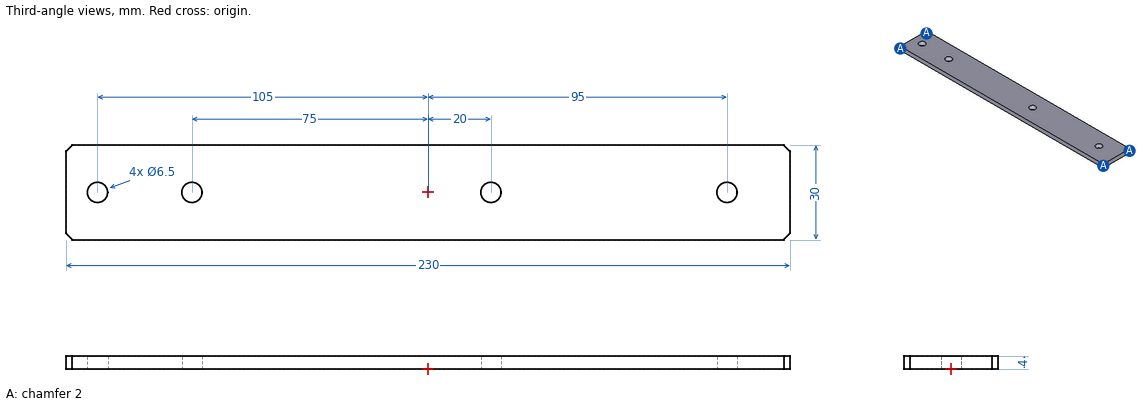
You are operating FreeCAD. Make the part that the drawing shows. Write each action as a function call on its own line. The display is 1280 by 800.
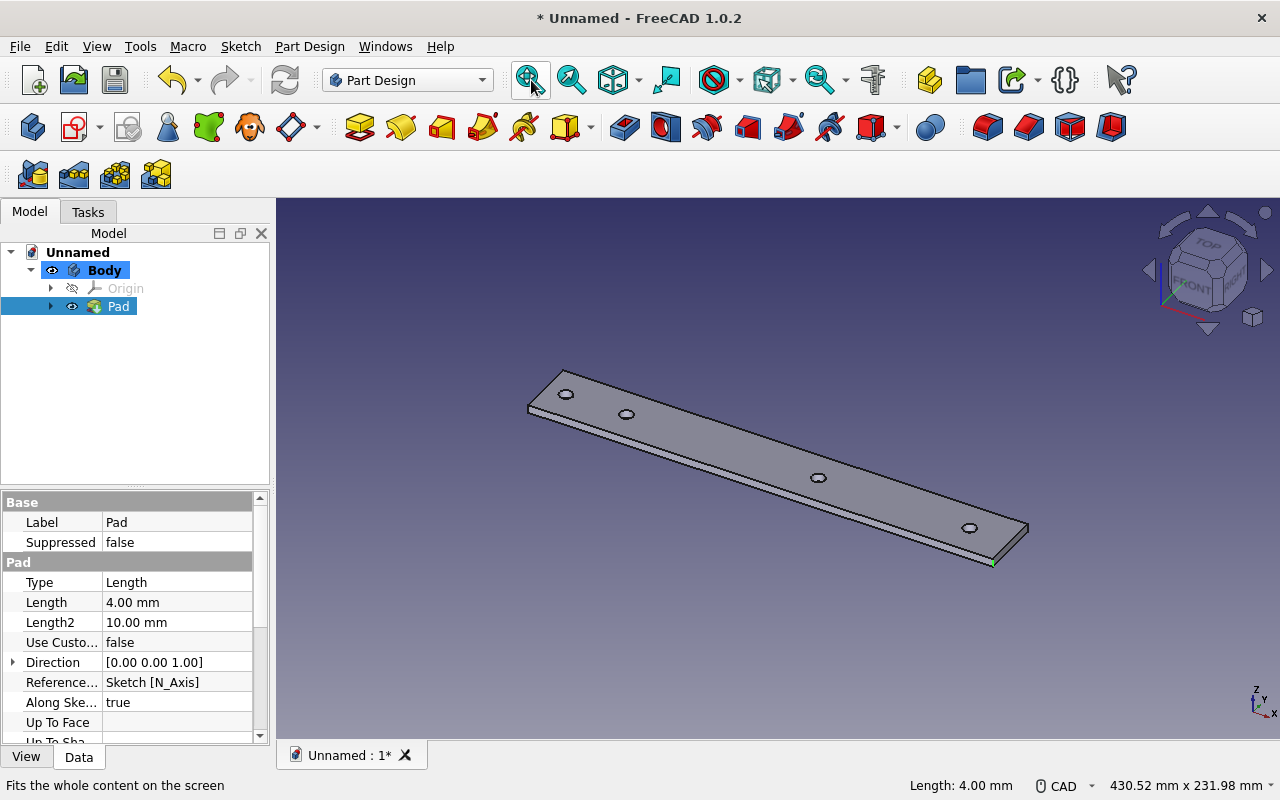
key(0)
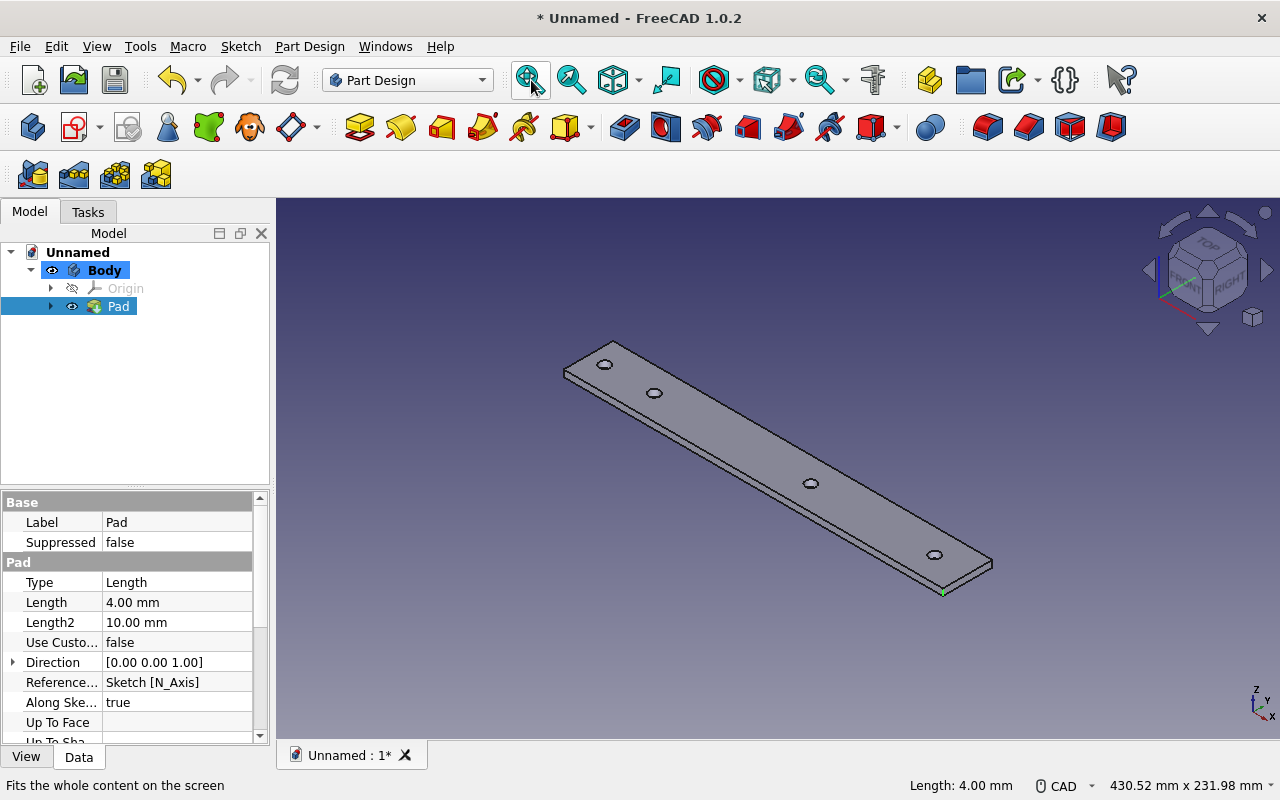
scroll(613, 344, up, 8)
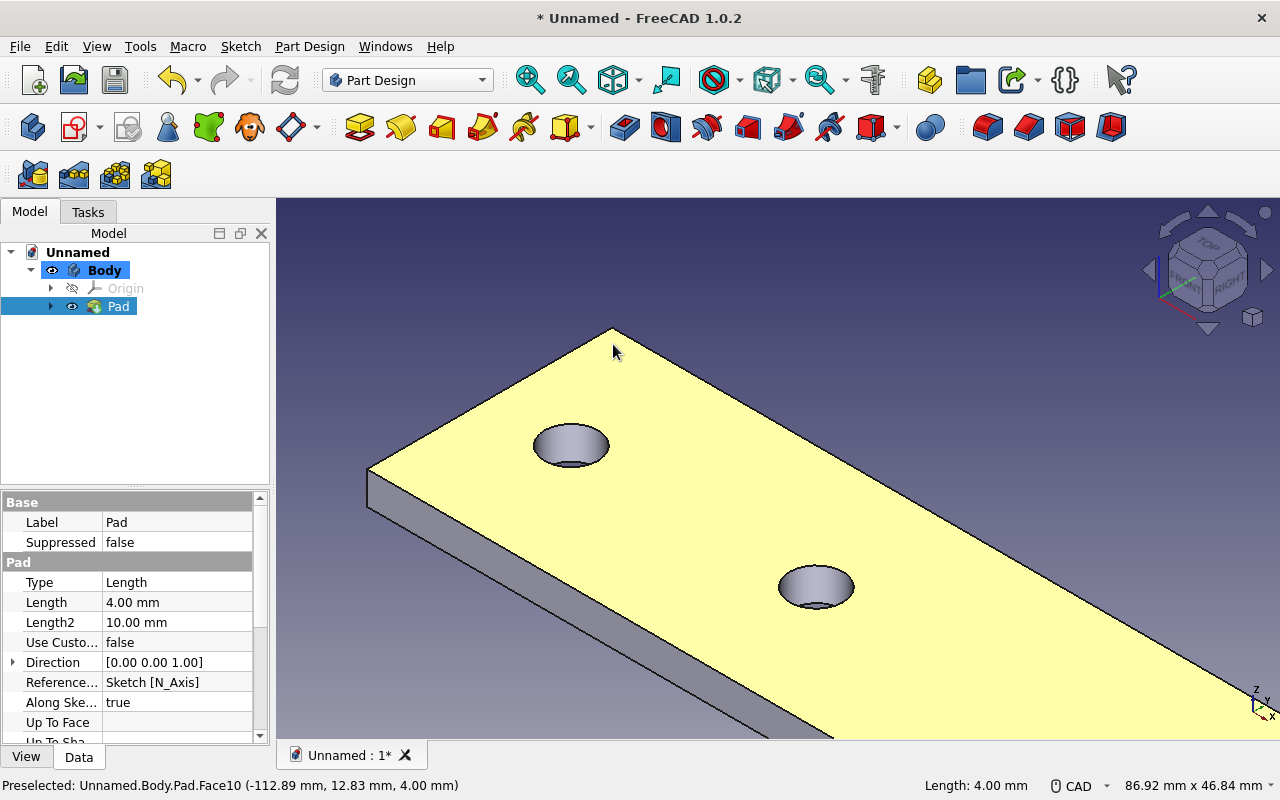
click(531, 80)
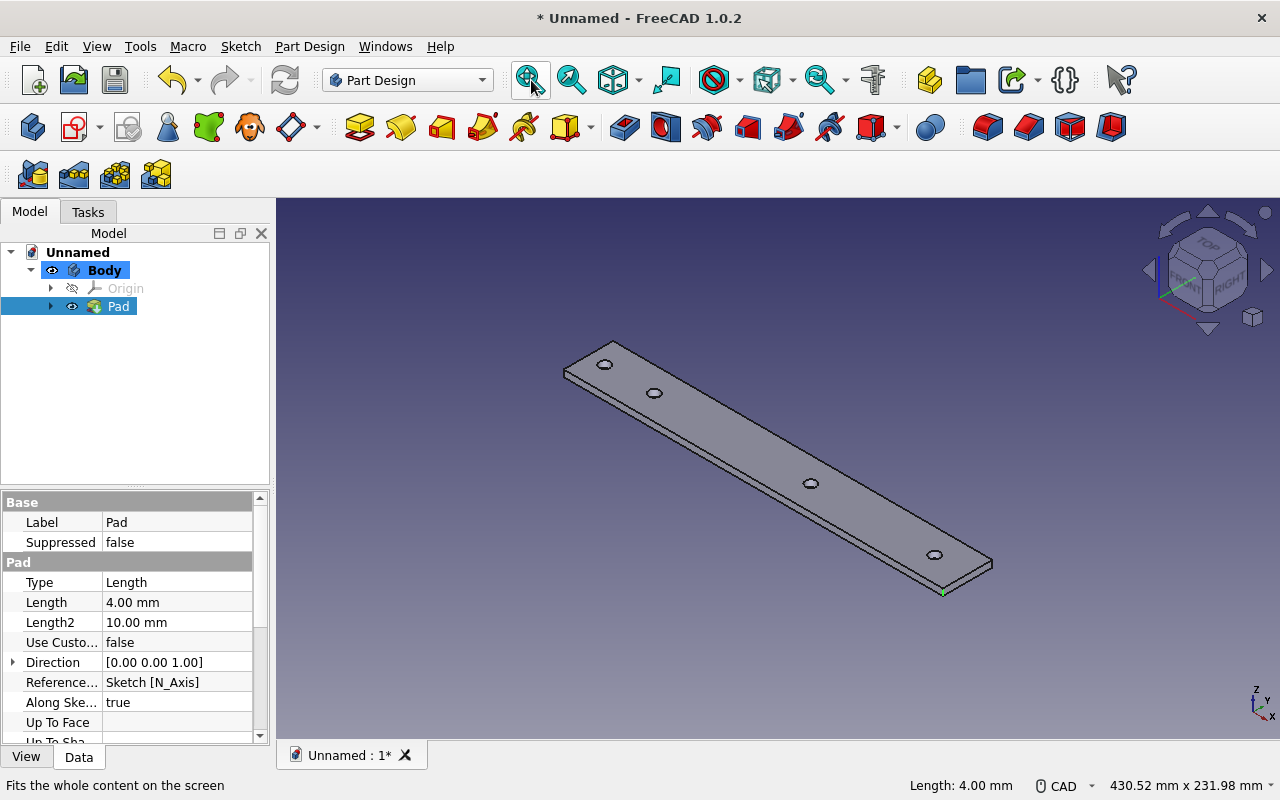
key(2)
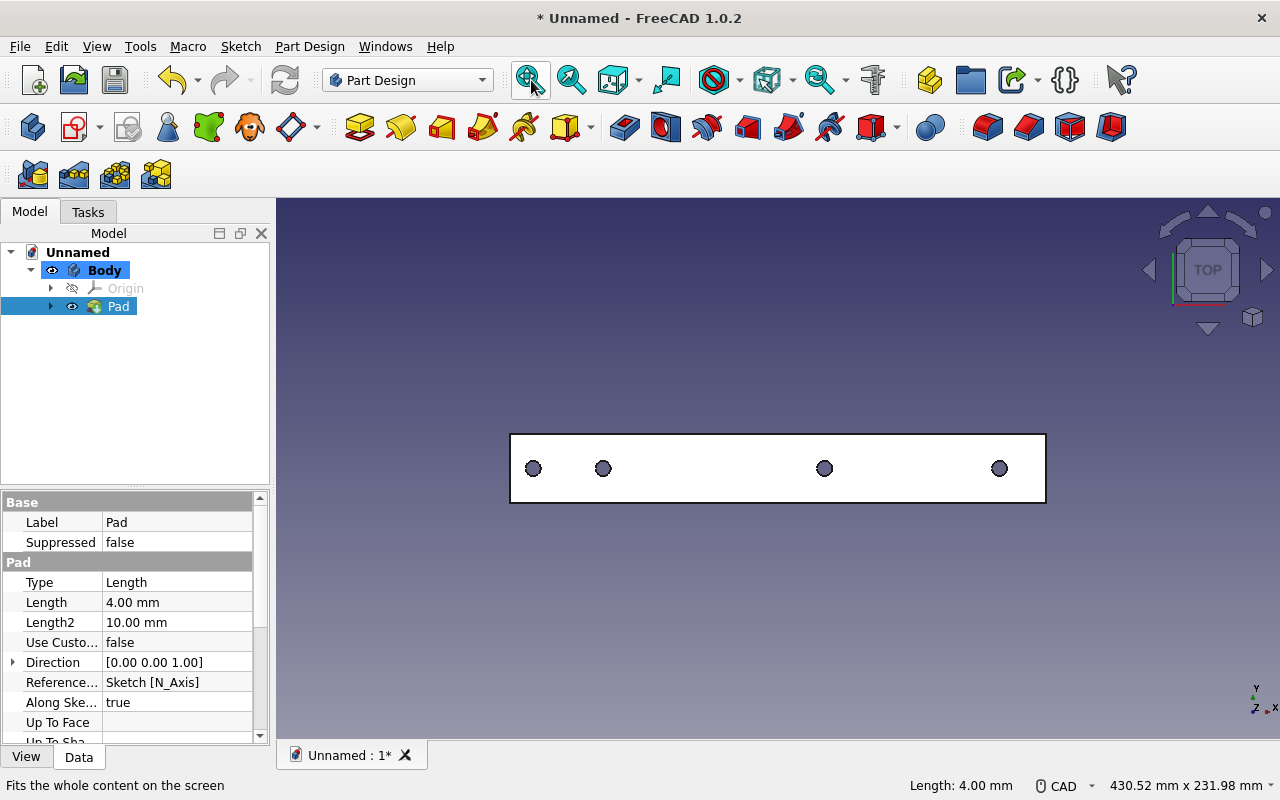
scroll(510, 433, up, 8)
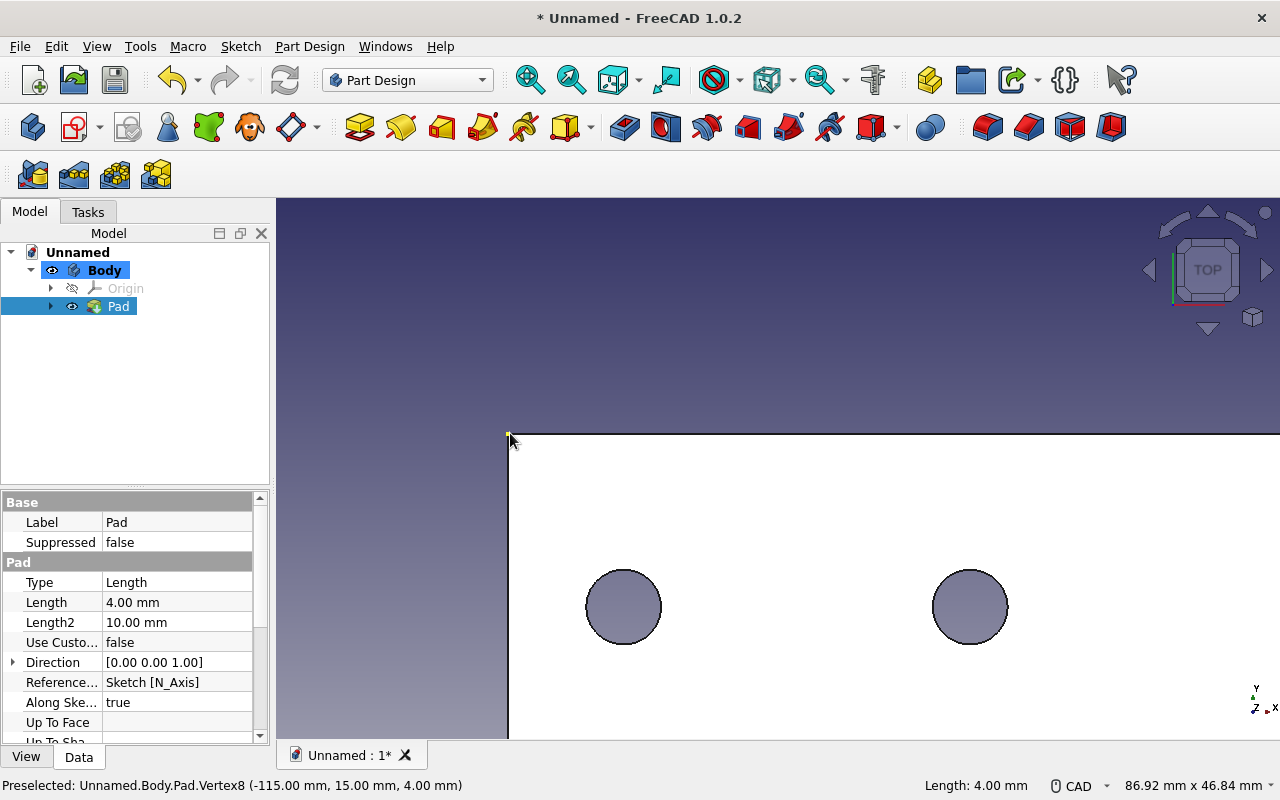
key(v)
key(f)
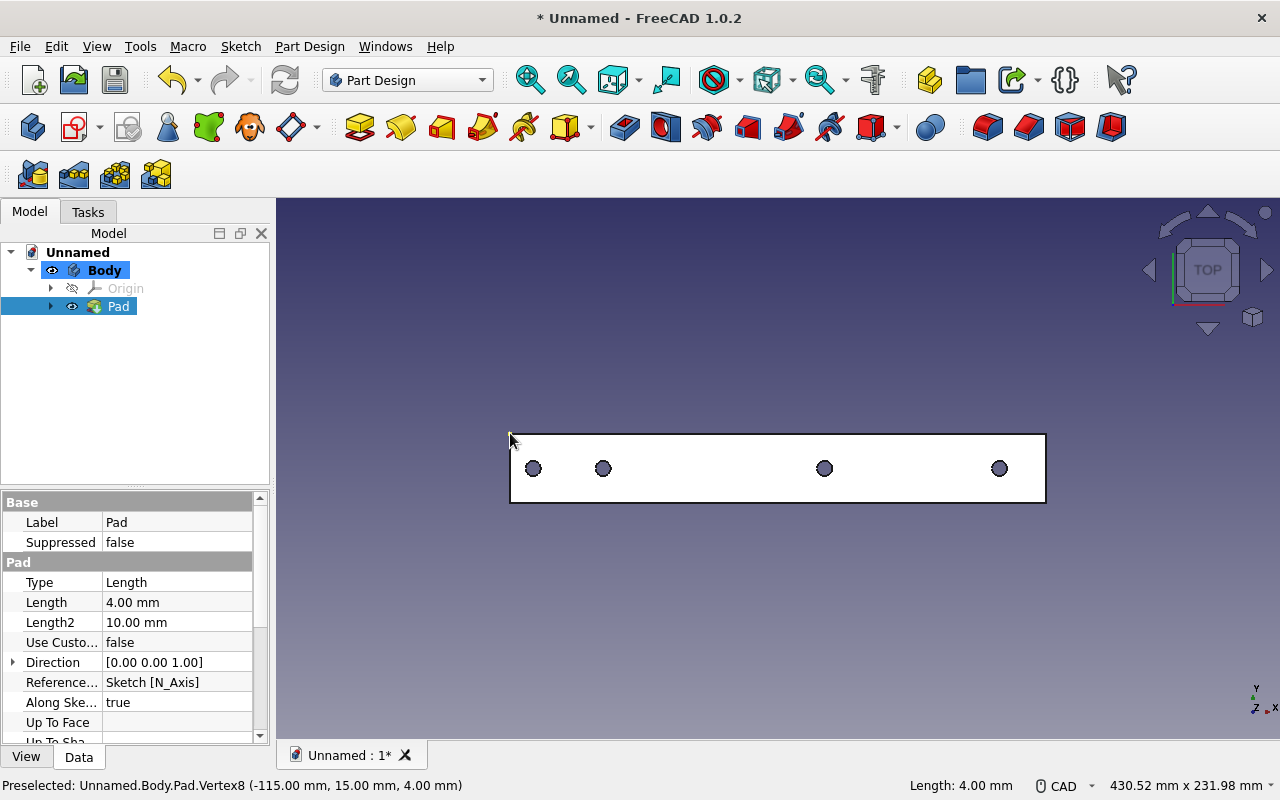
key(1)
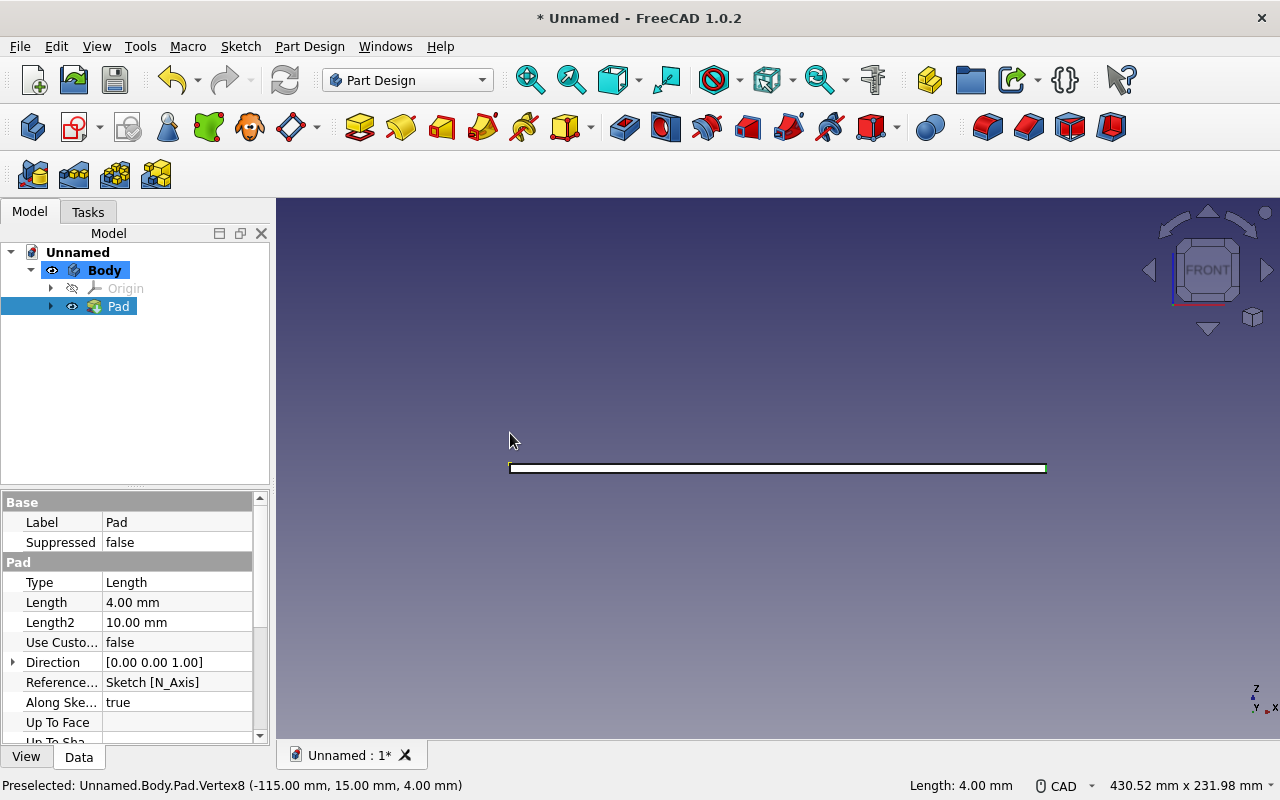
scroll(510, 468, up, 8)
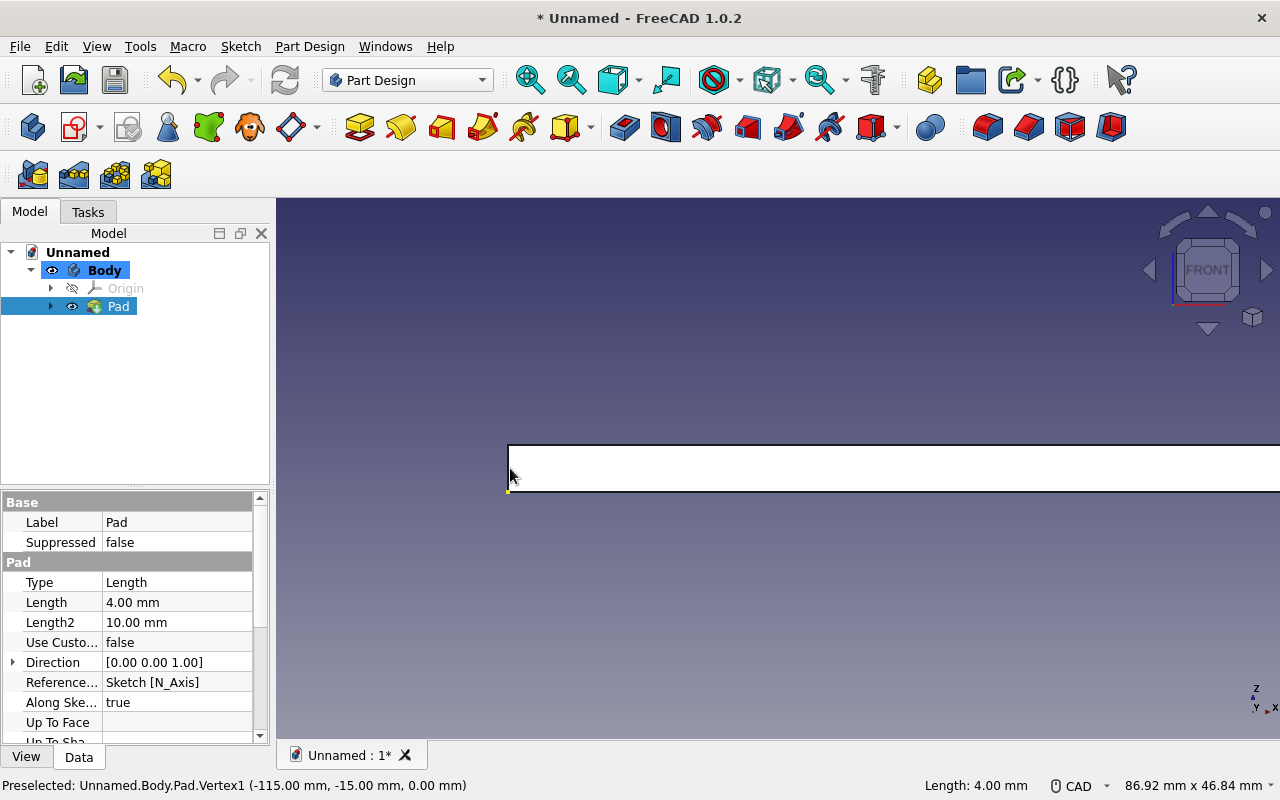
click(508, 468, ctrl)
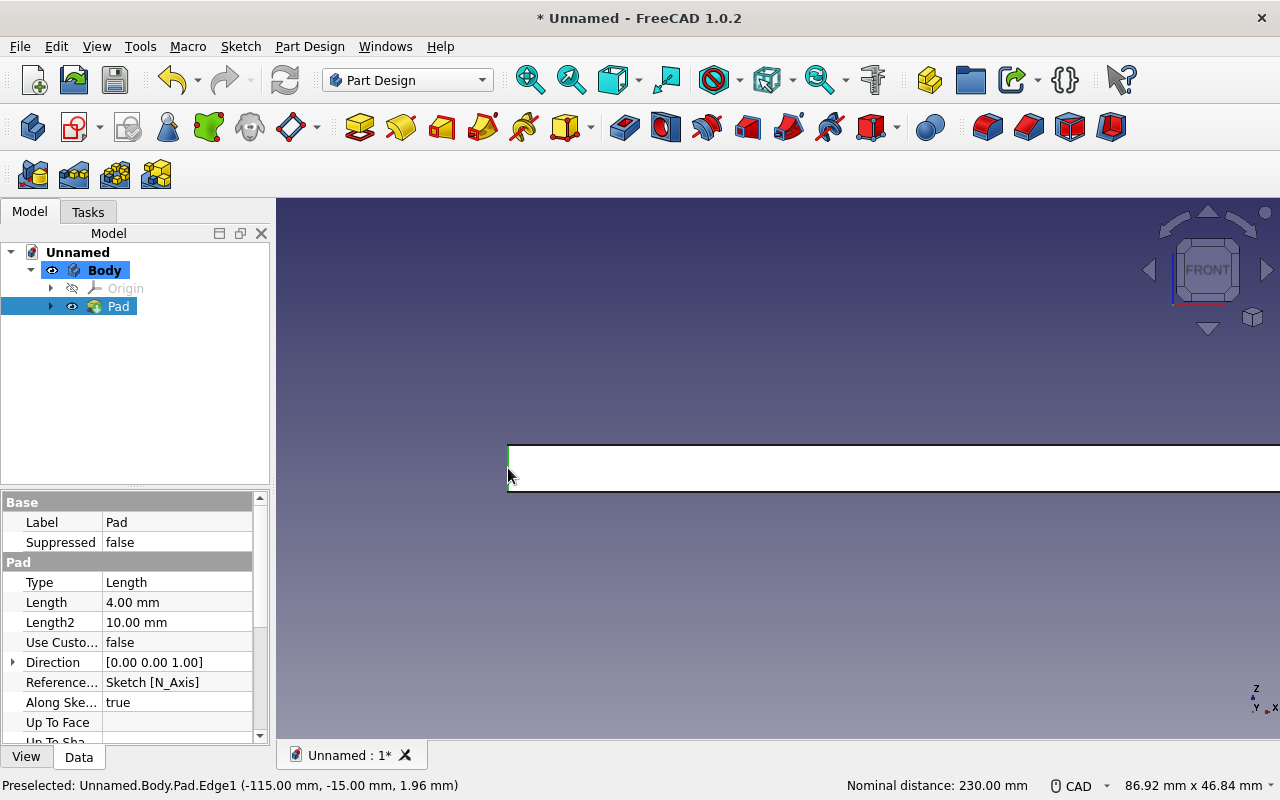
click(531, 80)